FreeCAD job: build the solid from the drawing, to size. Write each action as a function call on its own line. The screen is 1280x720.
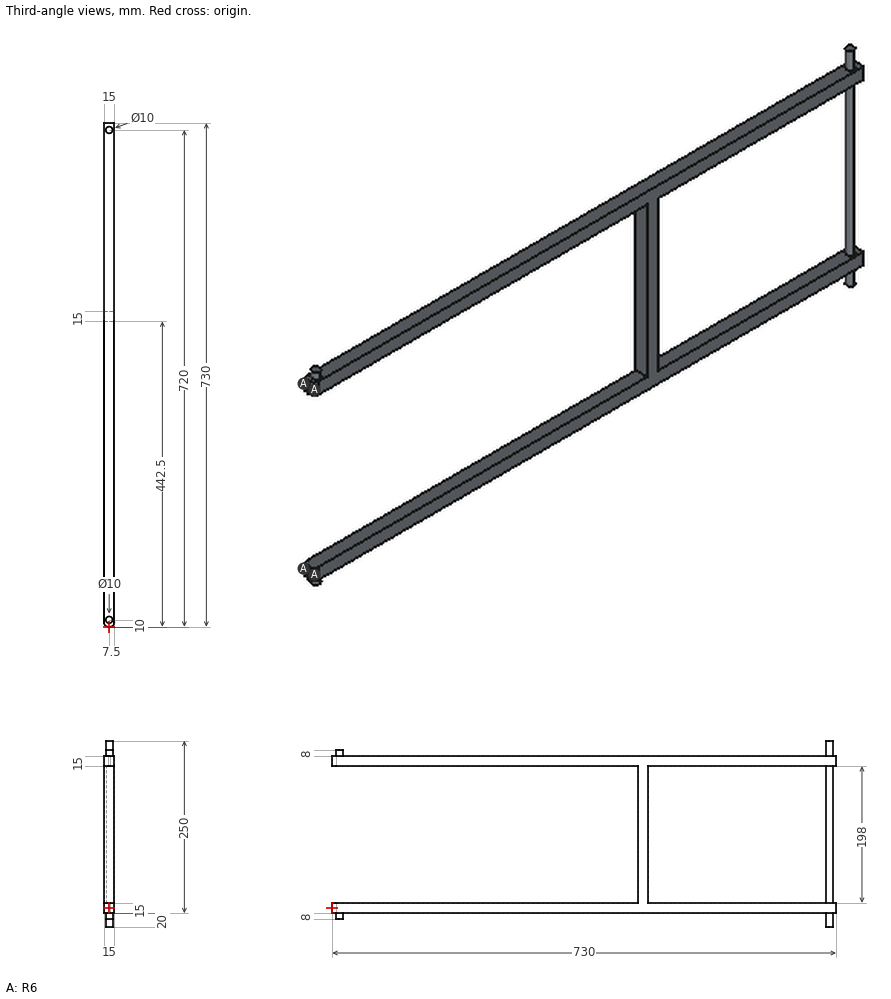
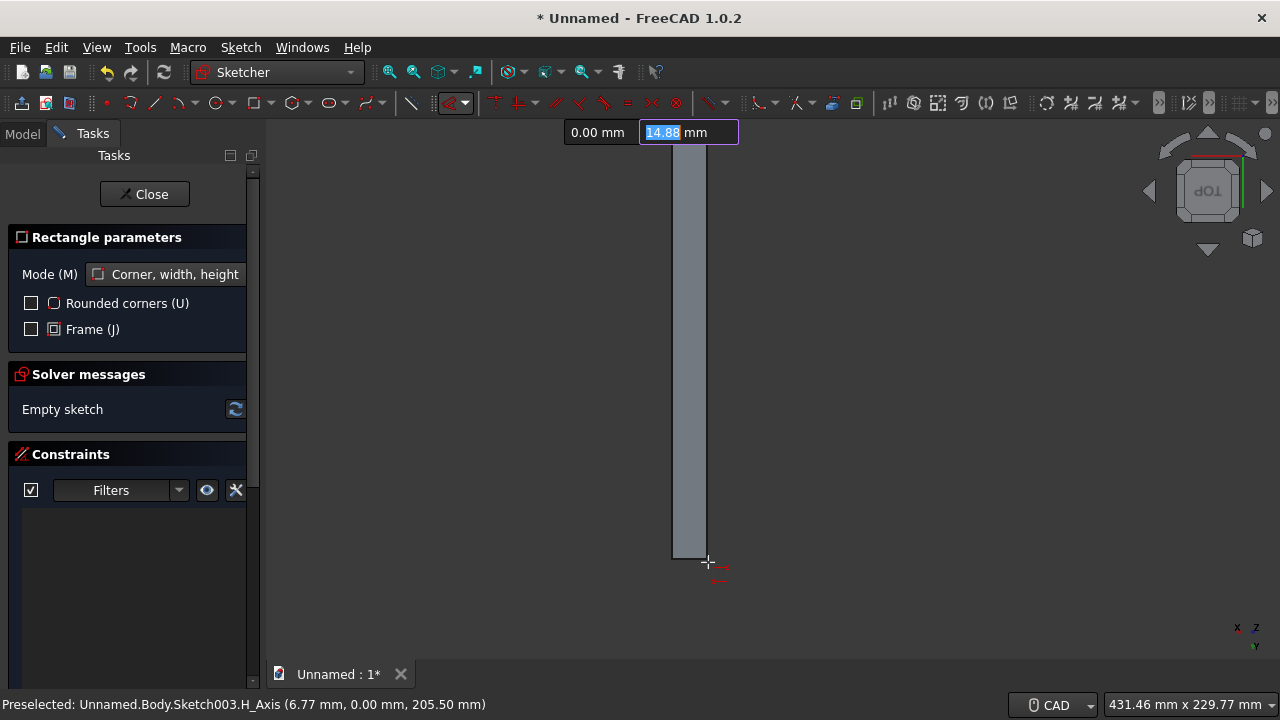
click(707, 559)
key(Escape)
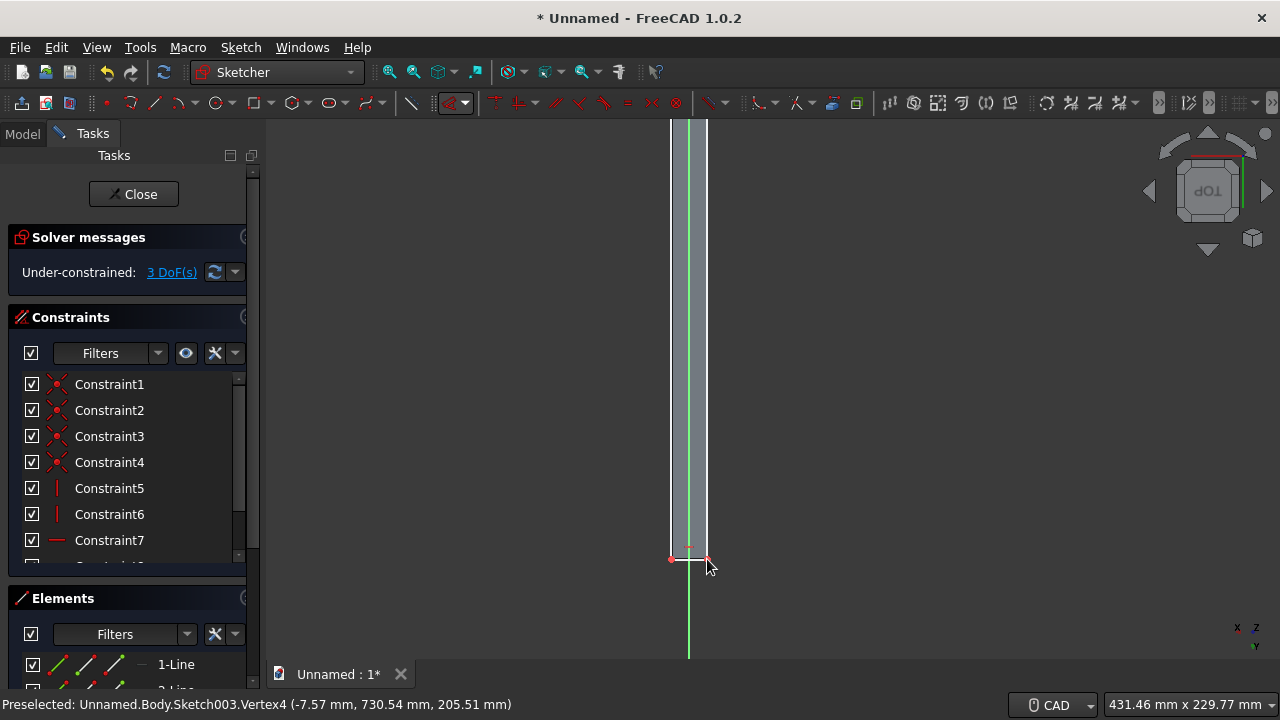
click(686, 560)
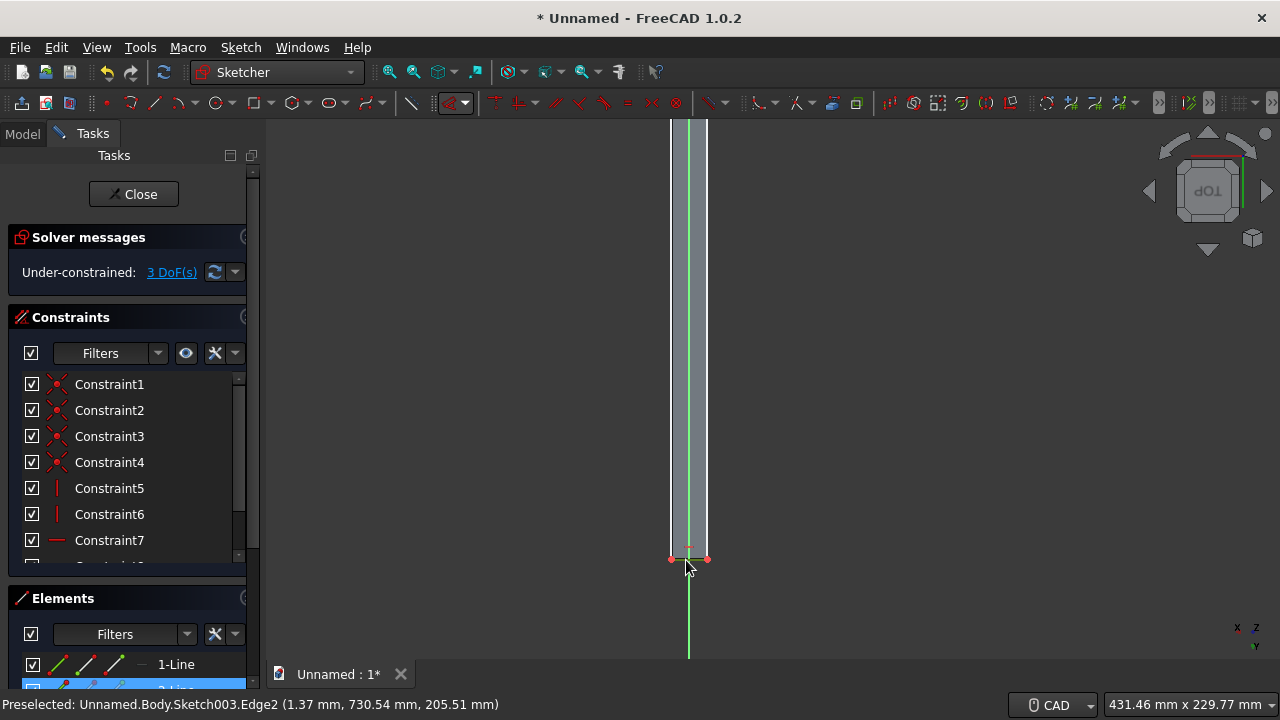
key(l)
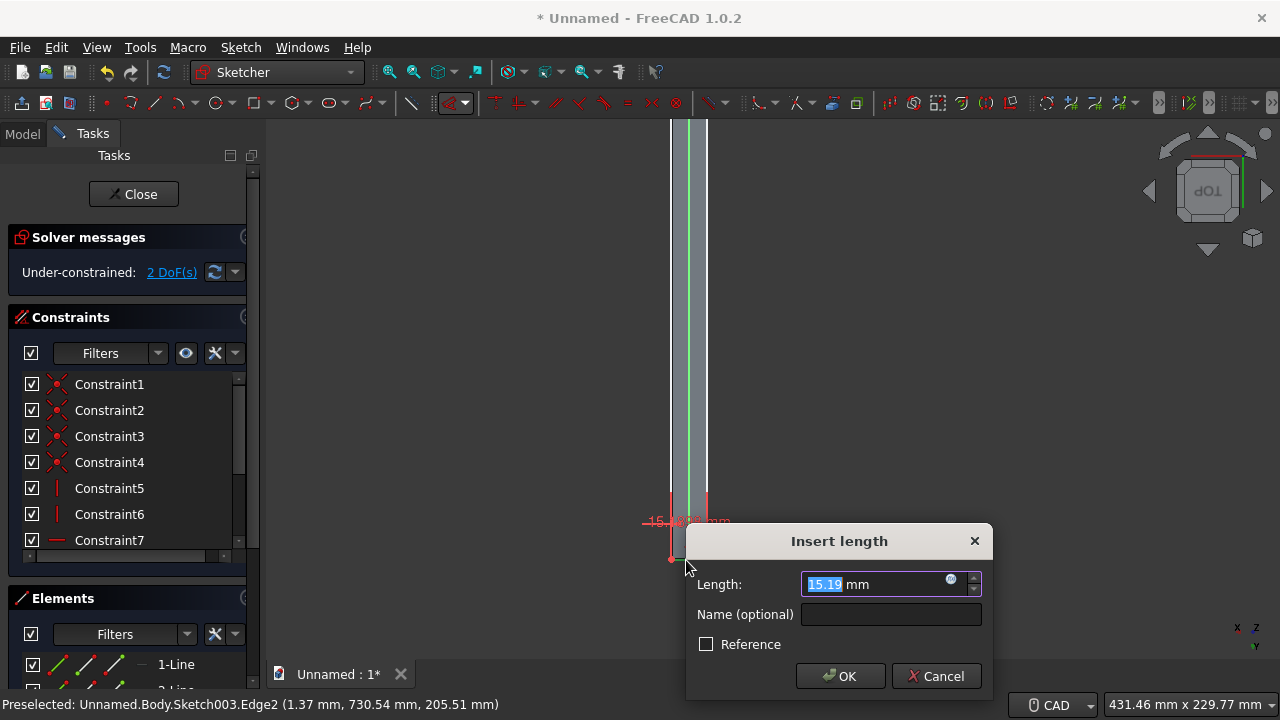
text(15)
key(Return)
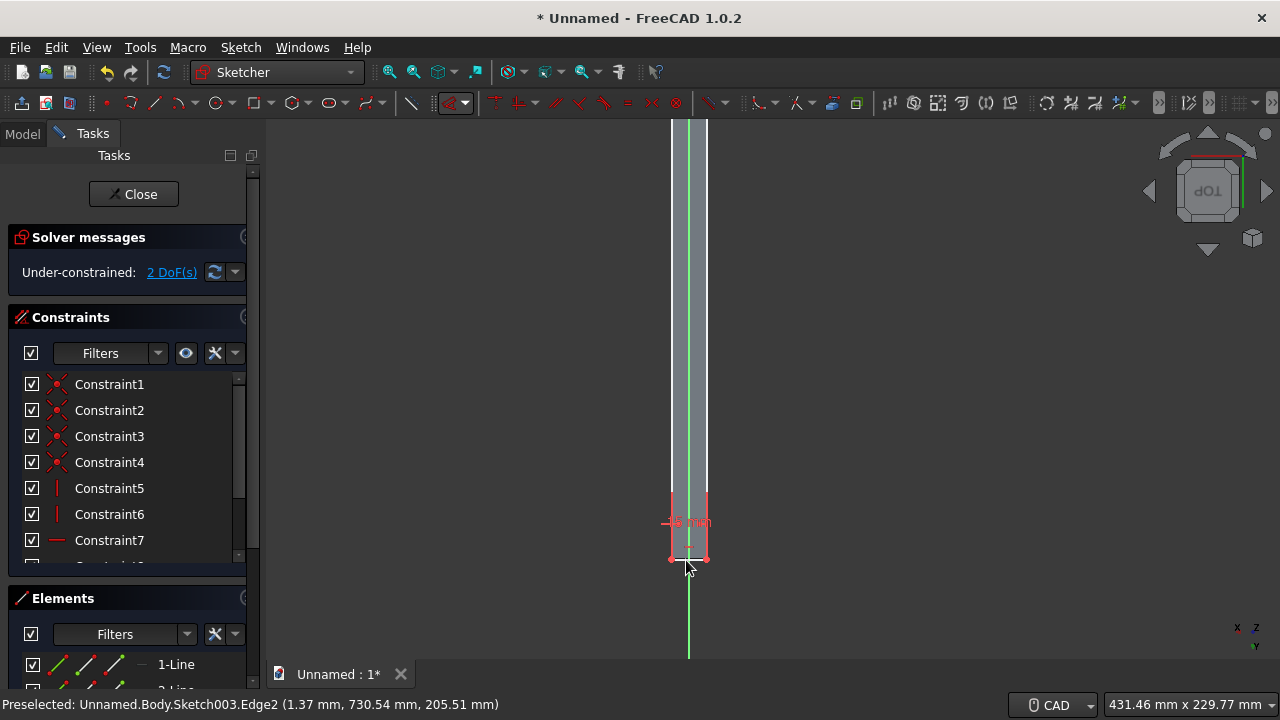
click(672, 217)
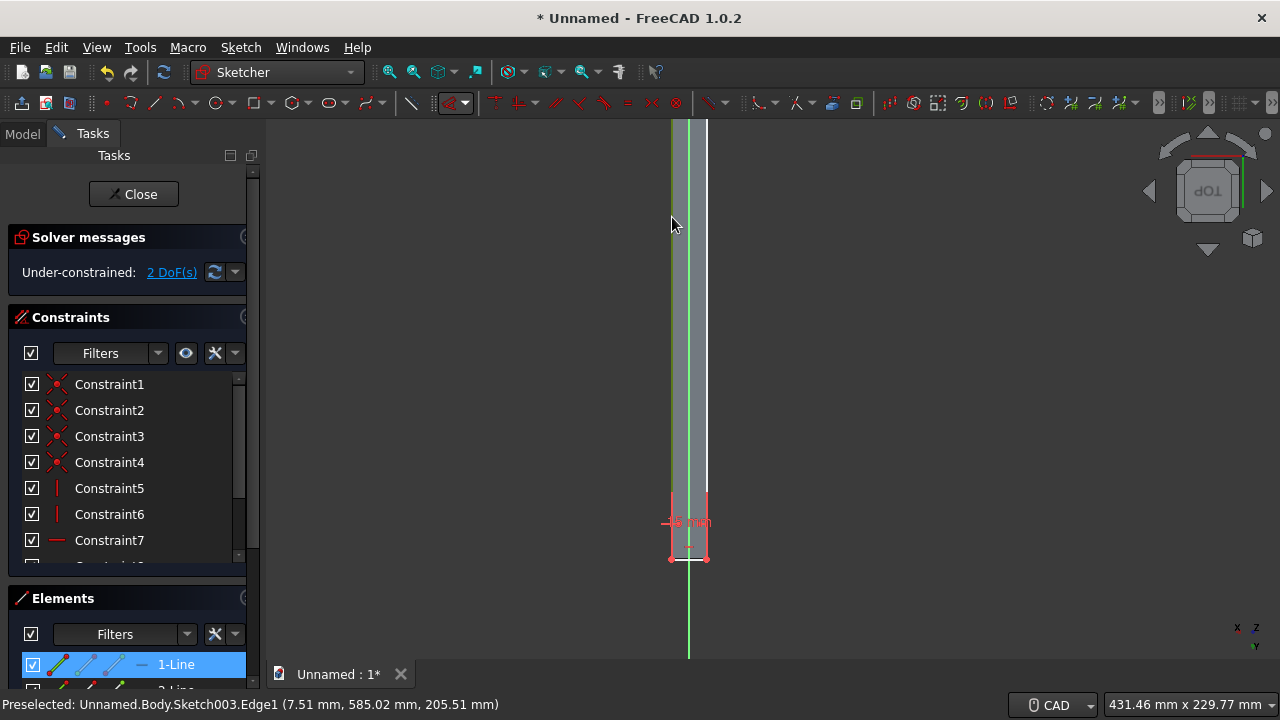
click(468, 104)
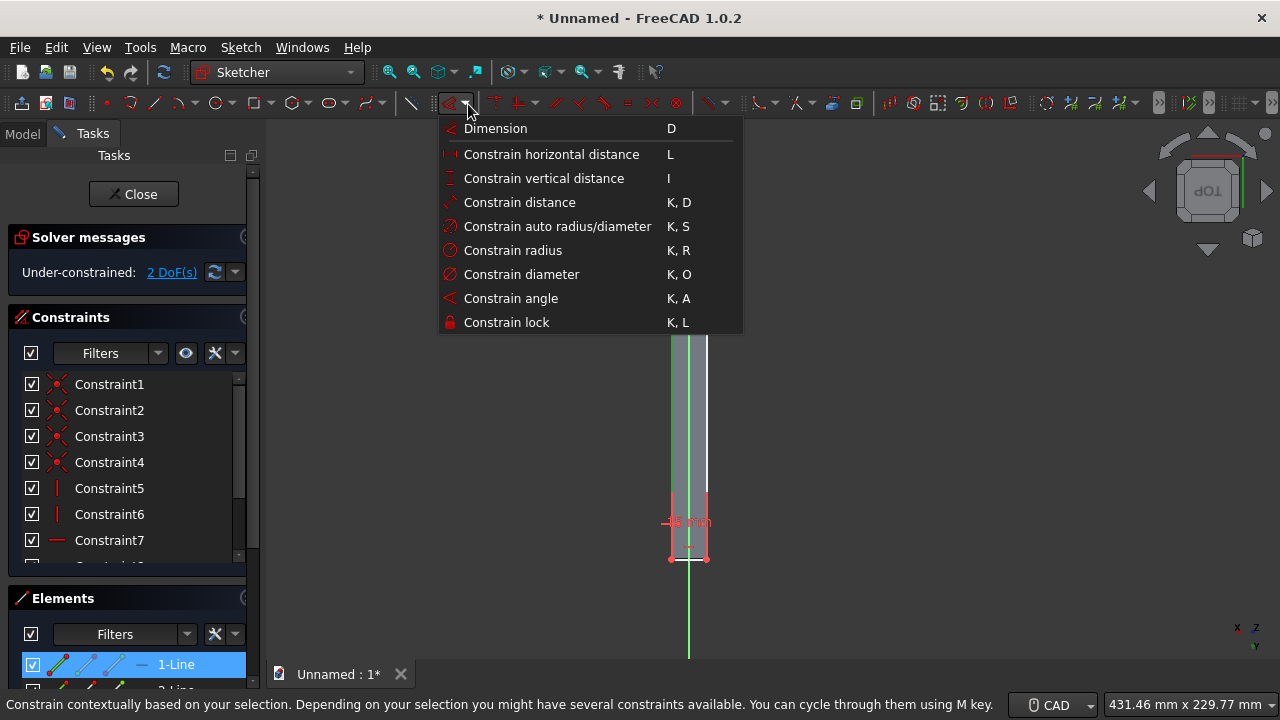
click(591, 178)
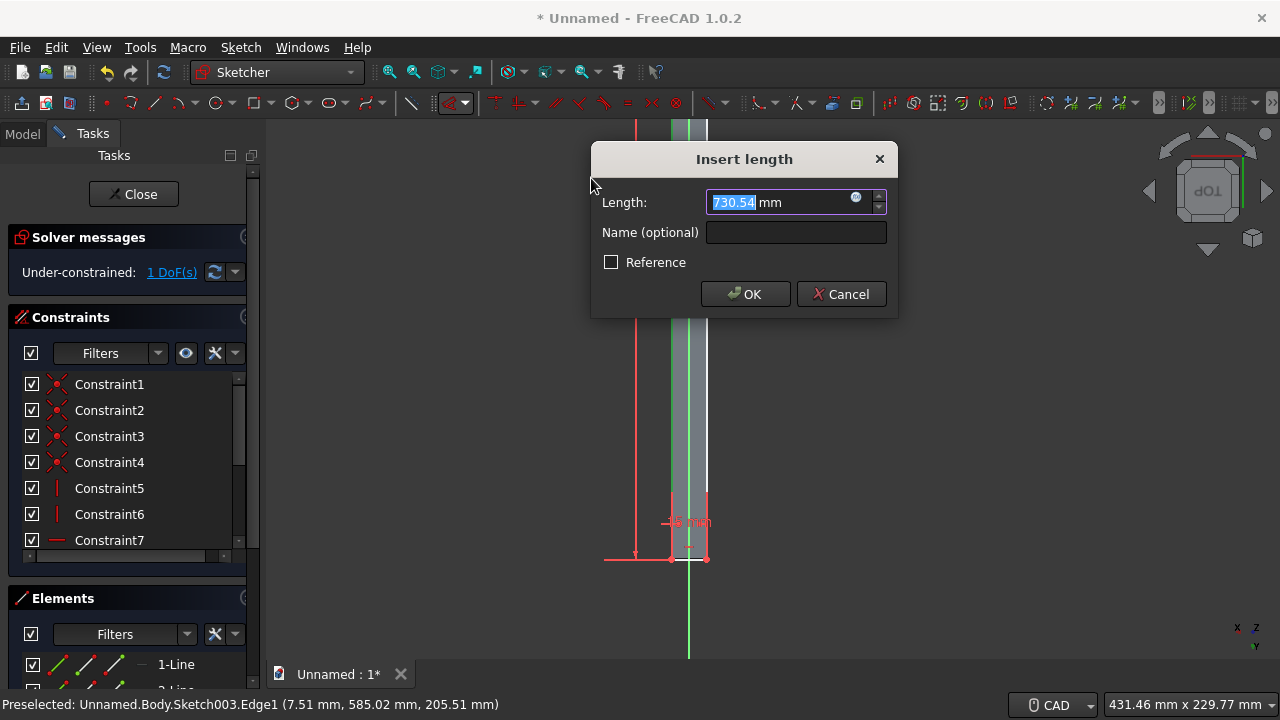
text(730)
key(Return)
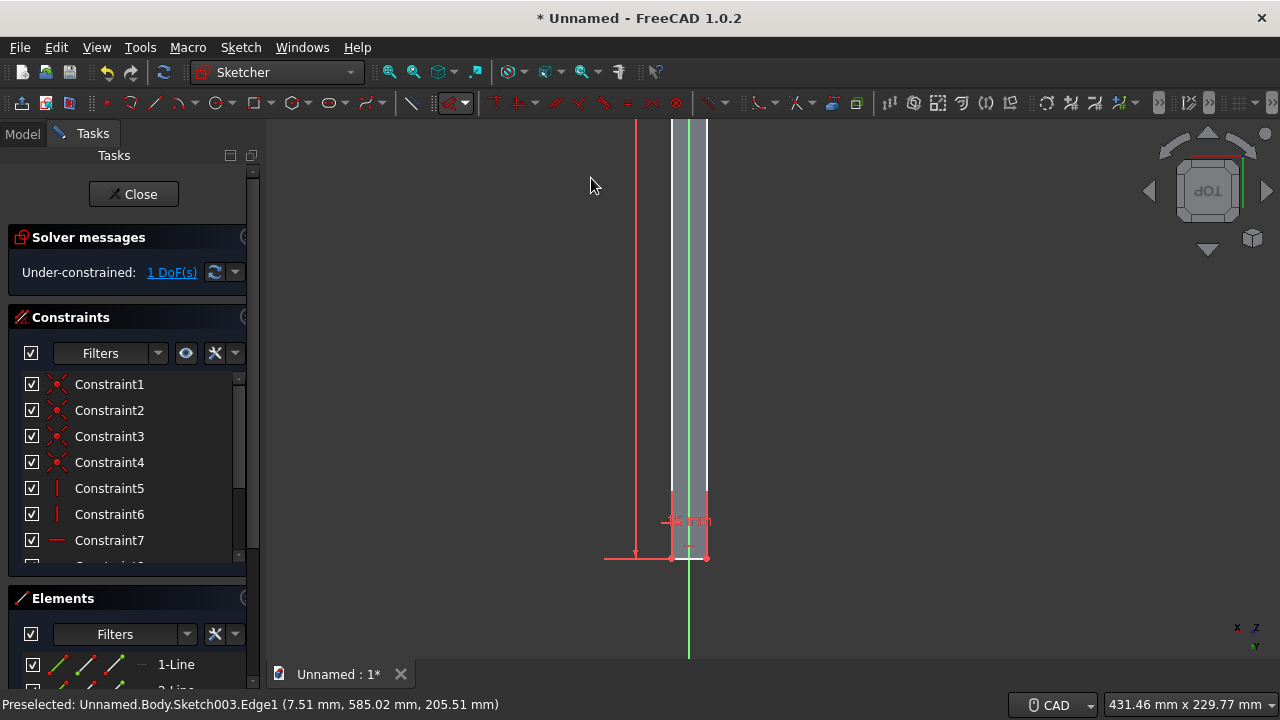
scroll(708, 563, down, 8)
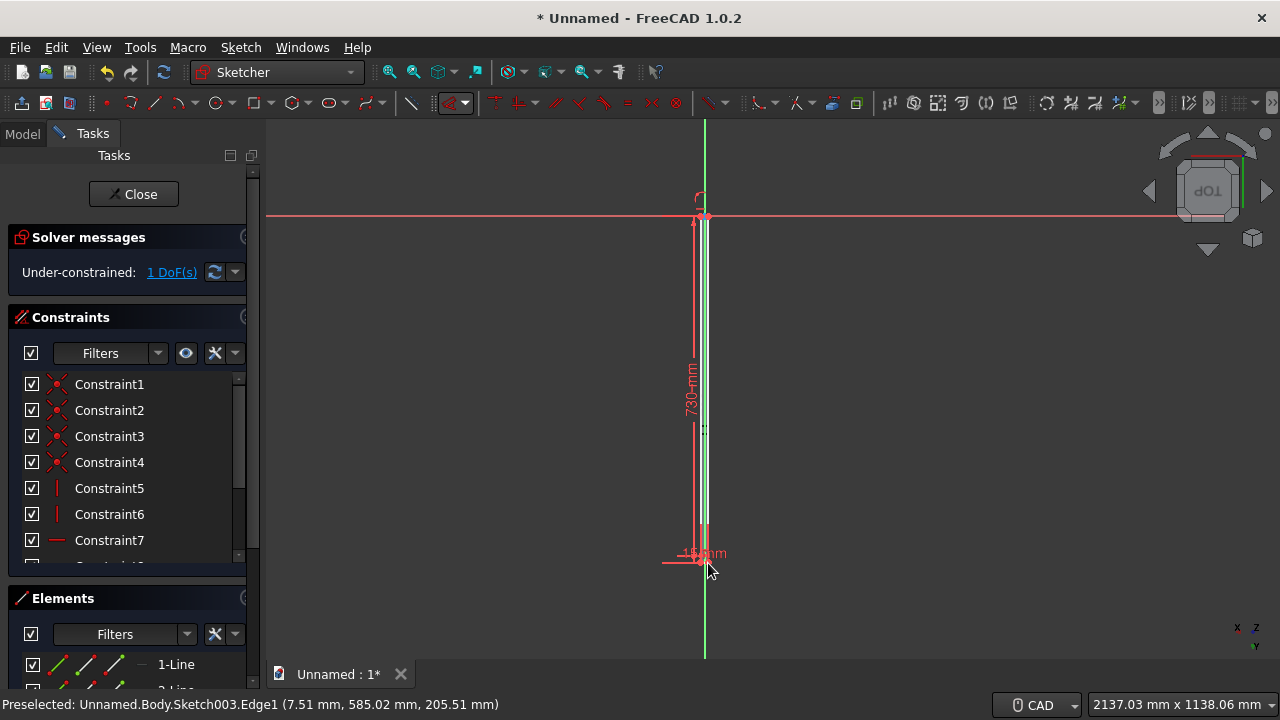
scroll(701, 216, up, 13)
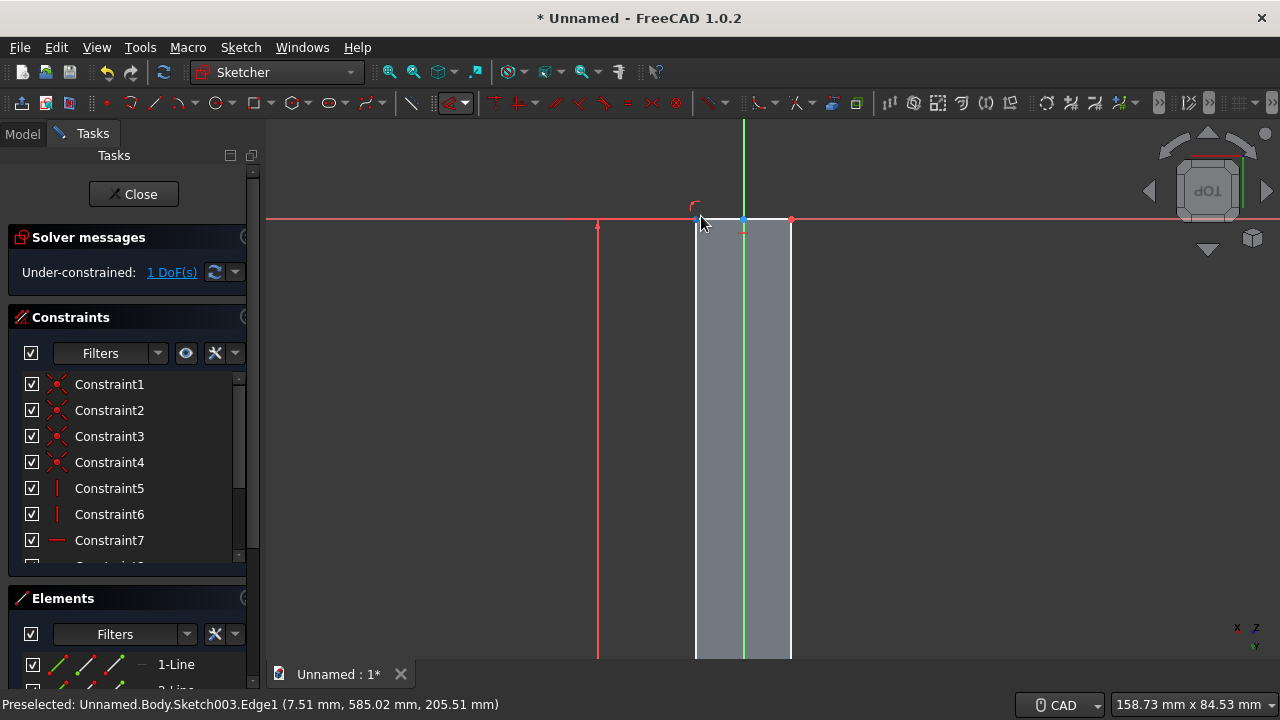
click(696, 219)